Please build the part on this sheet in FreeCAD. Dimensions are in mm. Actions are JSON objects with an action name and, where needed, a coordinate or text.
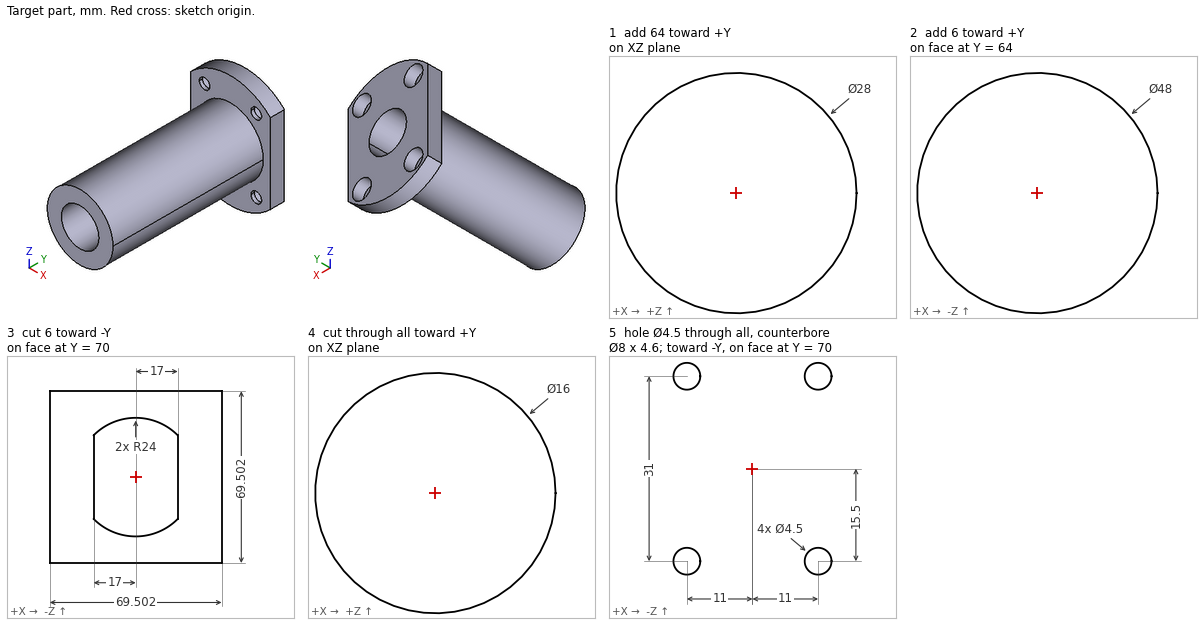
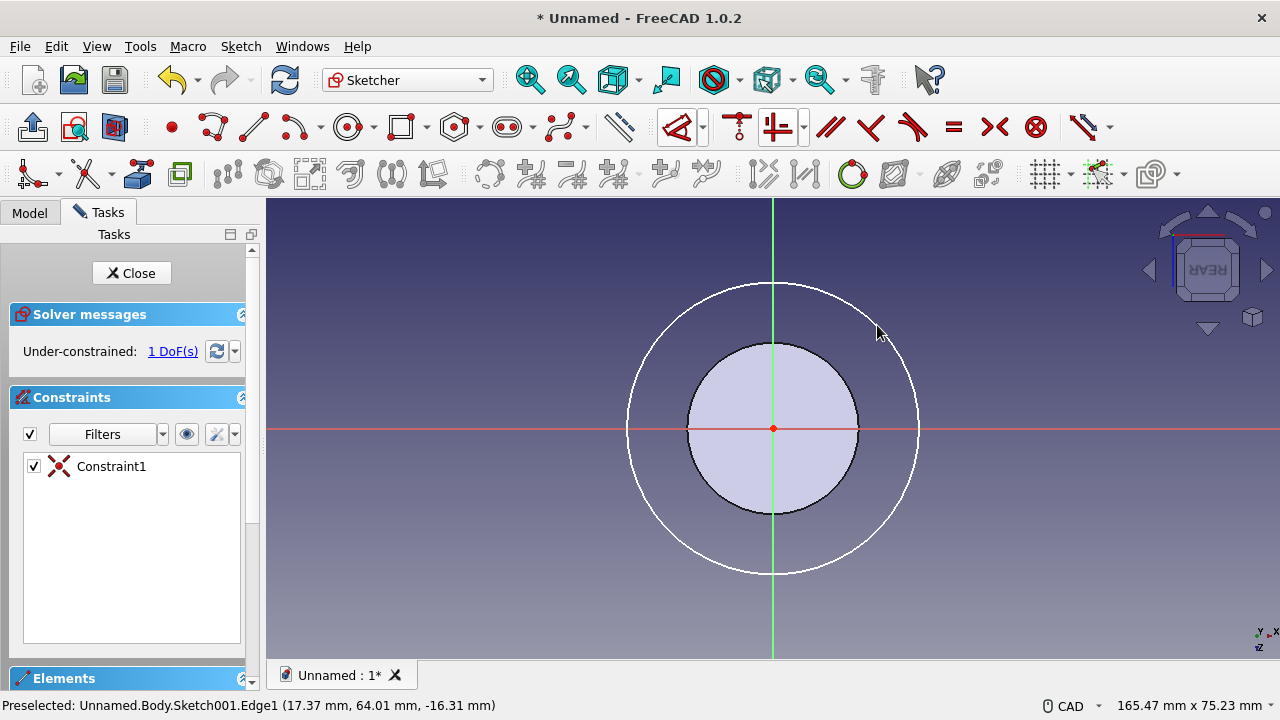
{"action": "left_click", "coordinate": [876, 325]}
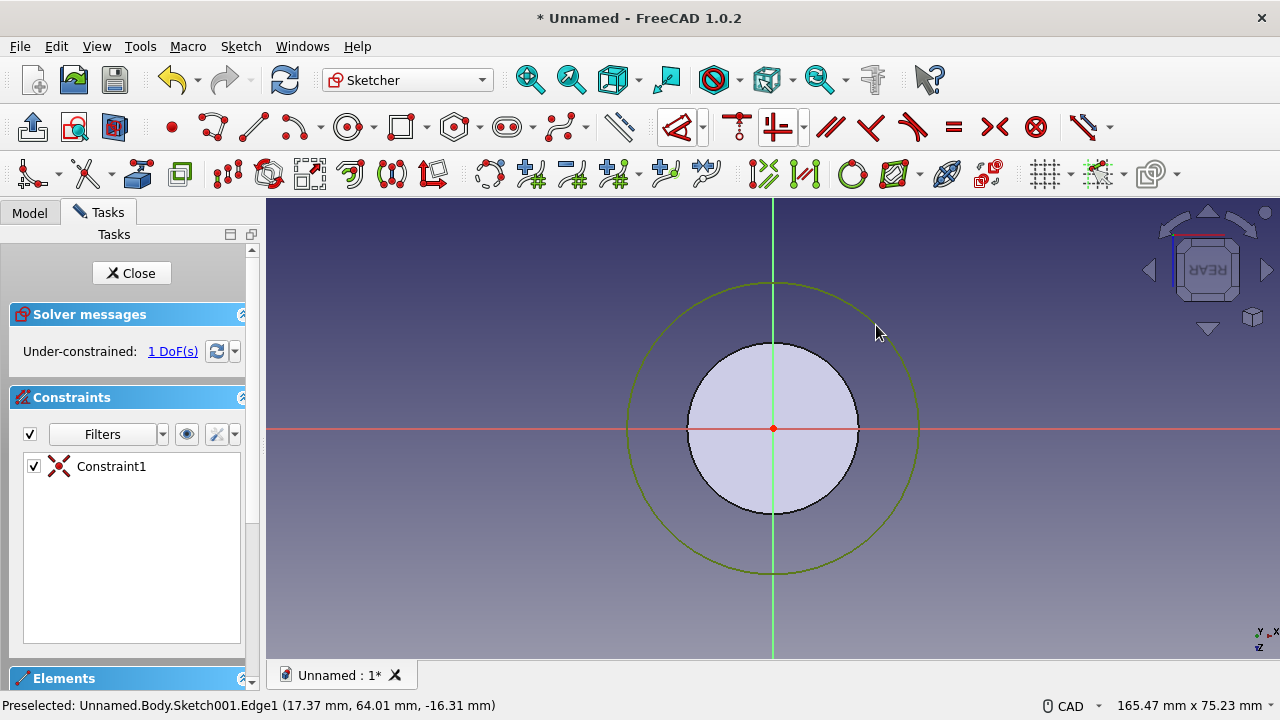
{"action": "key", "text": "k o"}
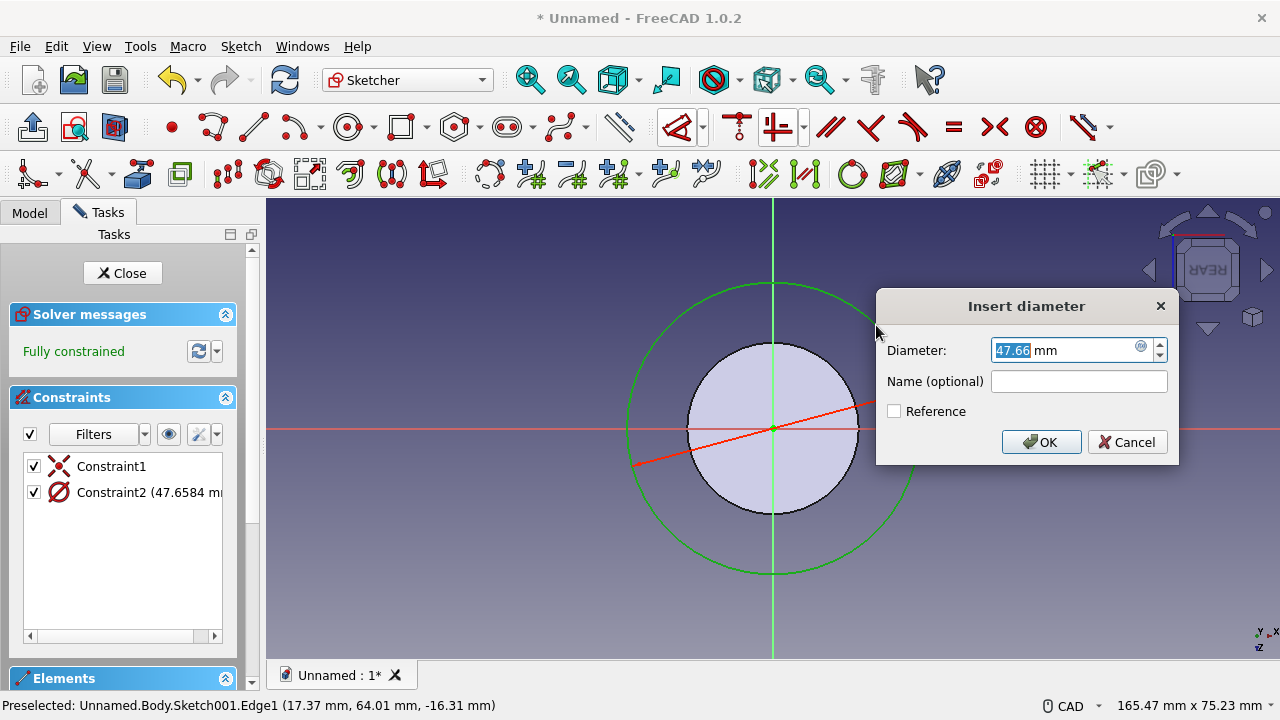
{"action": "type", "text": "48"}
{"action": "key", "text": "Return"}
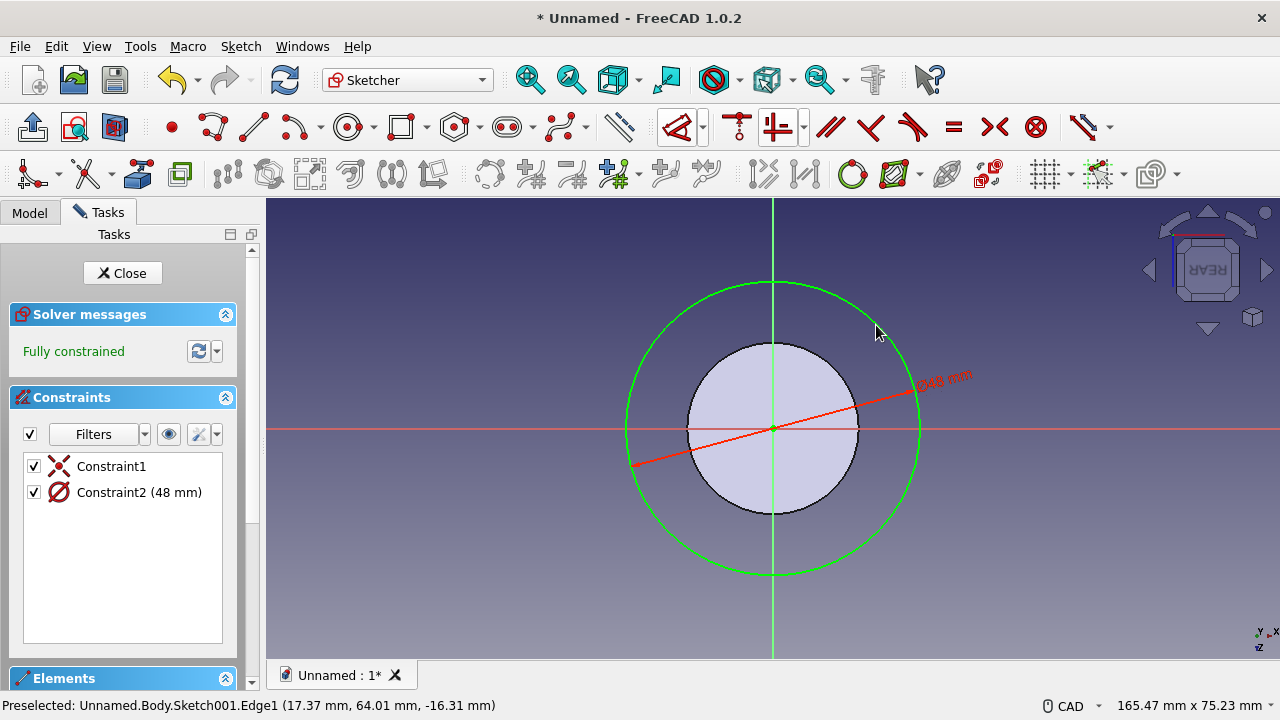
{"action": "left_click", "coordinate": [123, 273]}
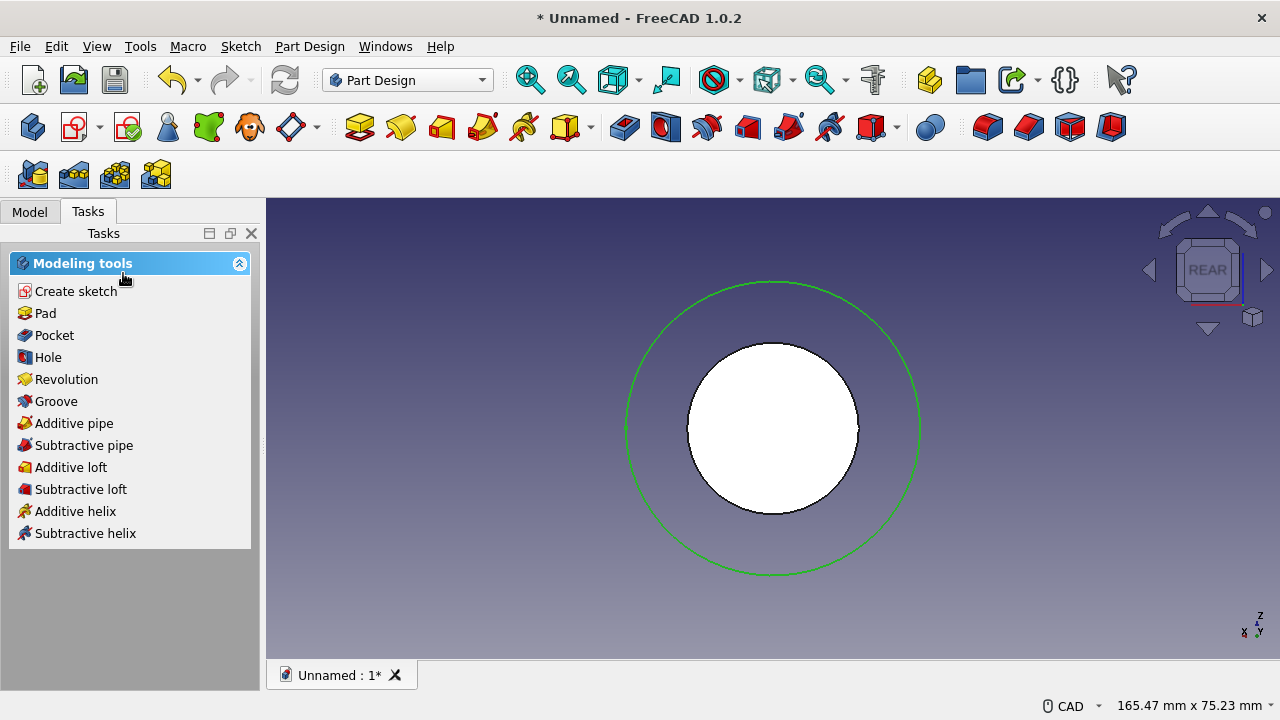
{"action": "left_click", "coordinate": [360, 128]}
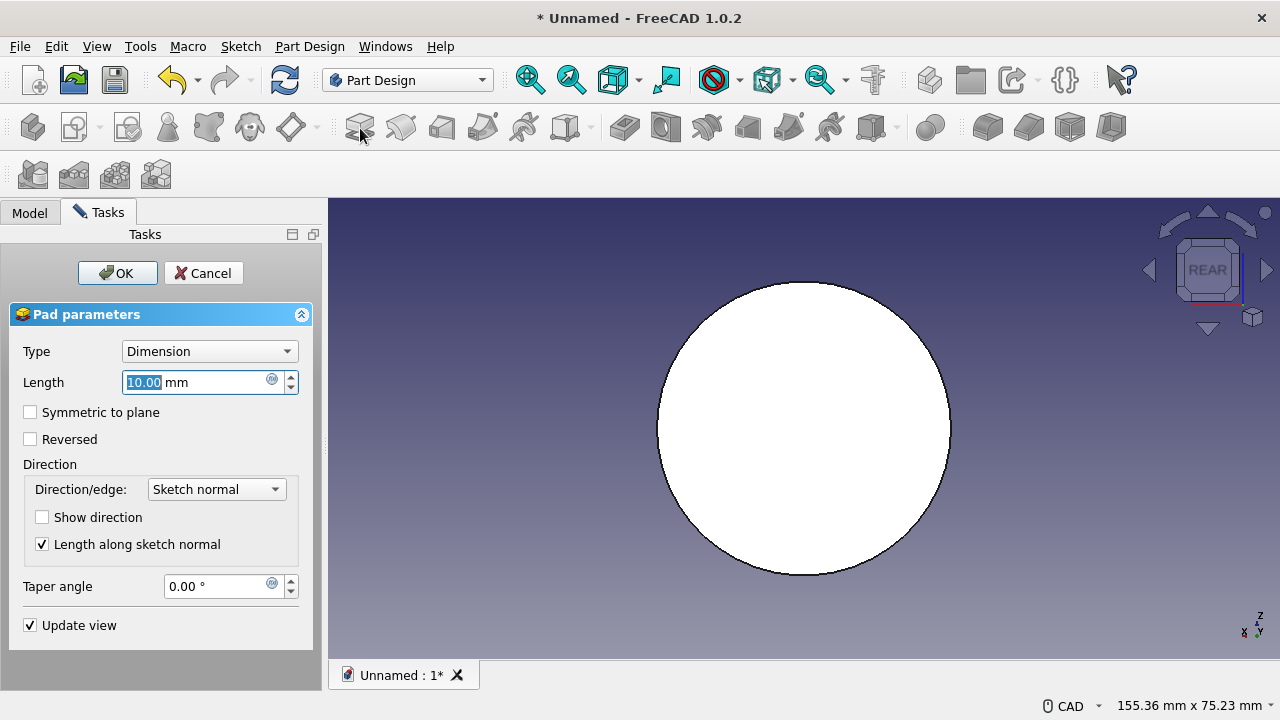
{"action": "type", "text": "6"}
{"action": "key", "text": "Tab"}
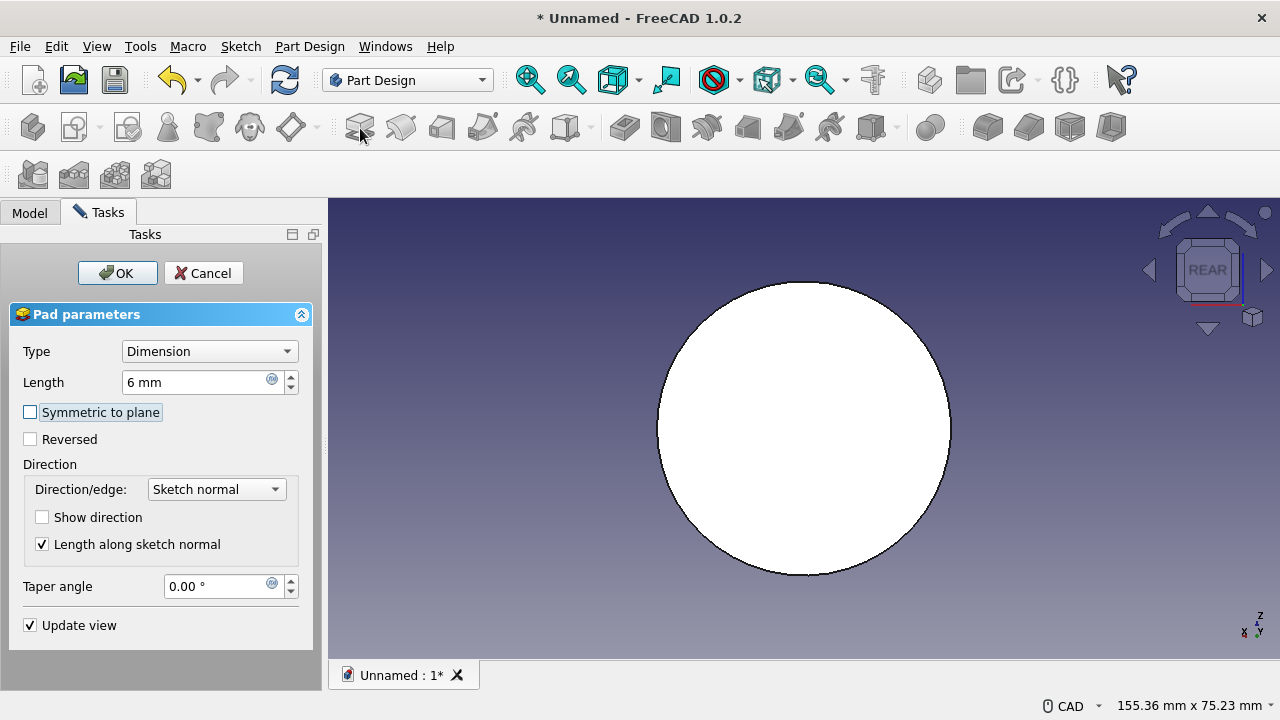
{"action": "left_click", "coordinate": [118, 273]}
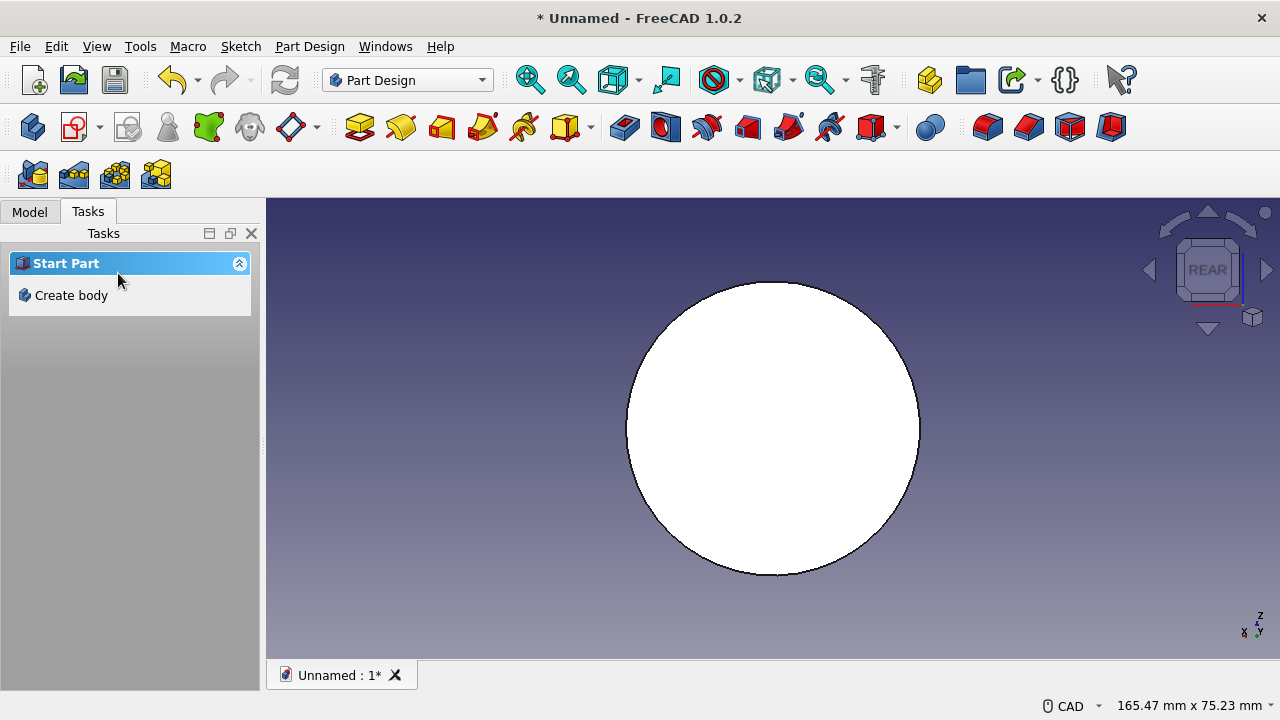
{"action": "left_click", "coordinate": [773, 428]}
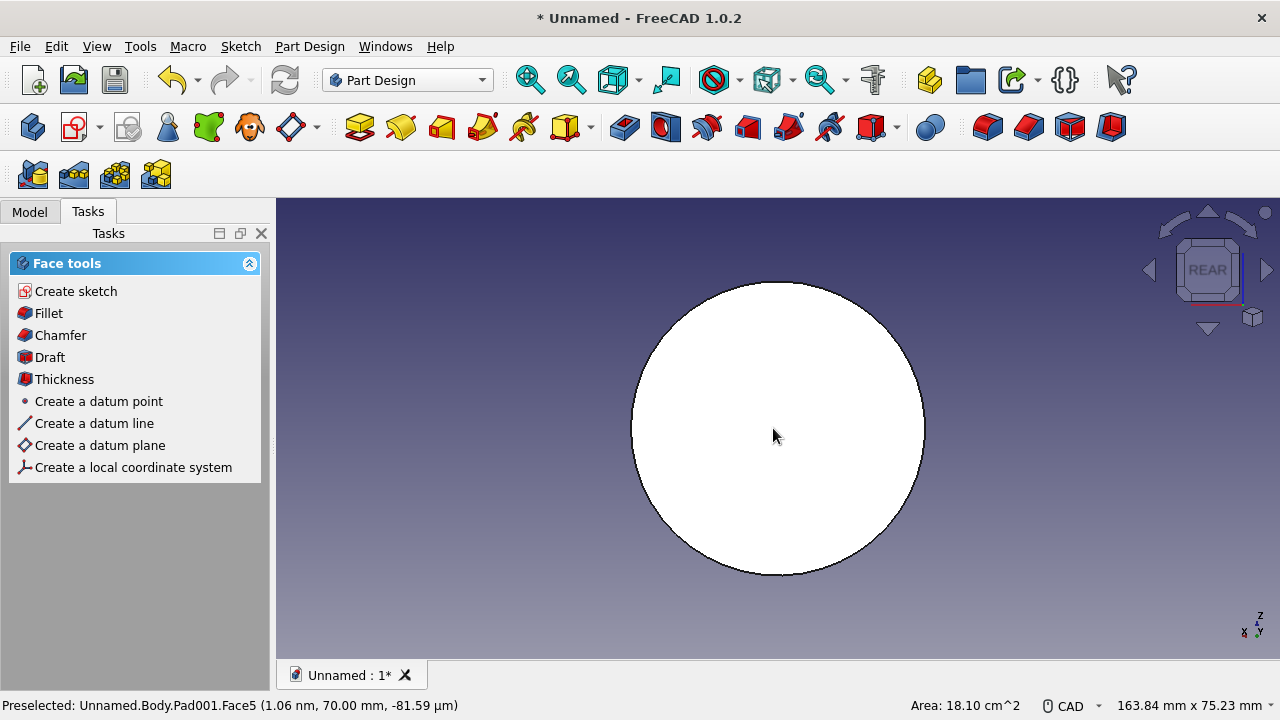
{"action": "left_click", "coordinate": [74, 128]}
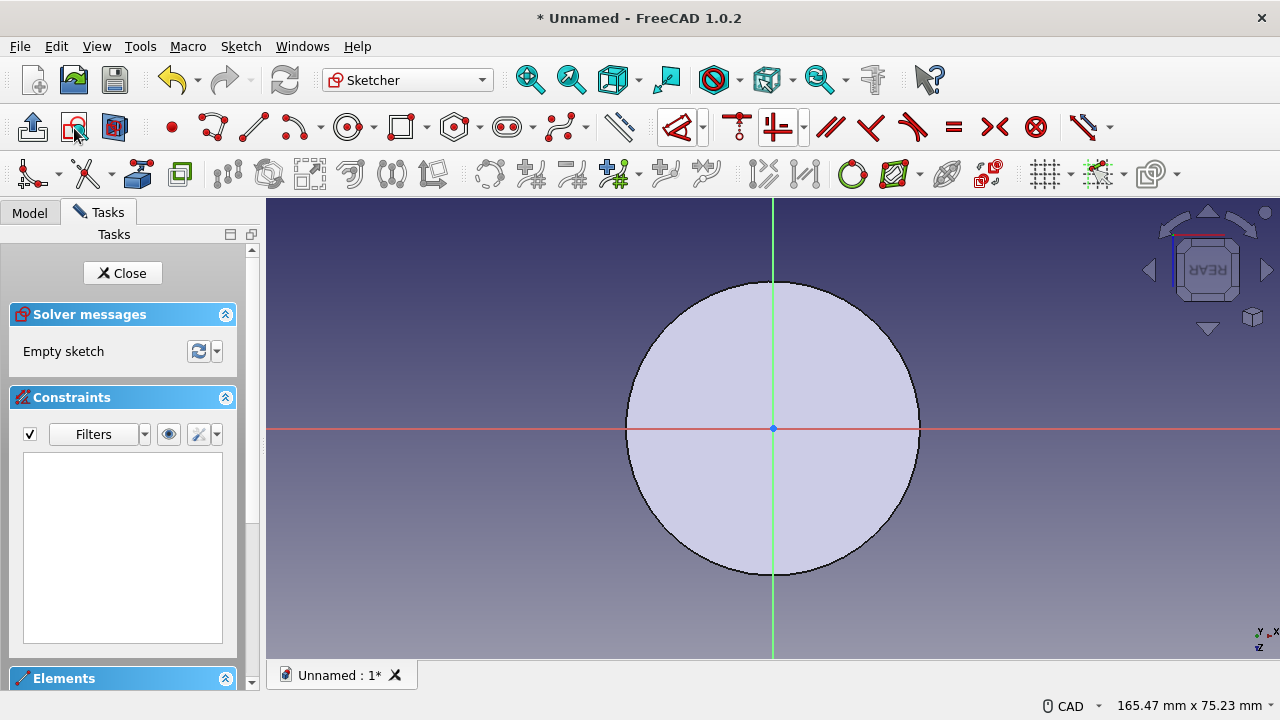
{"action": "scroll", "coordinate": [565, 429], "scroll_direction": "down", "scroll_amount": 2}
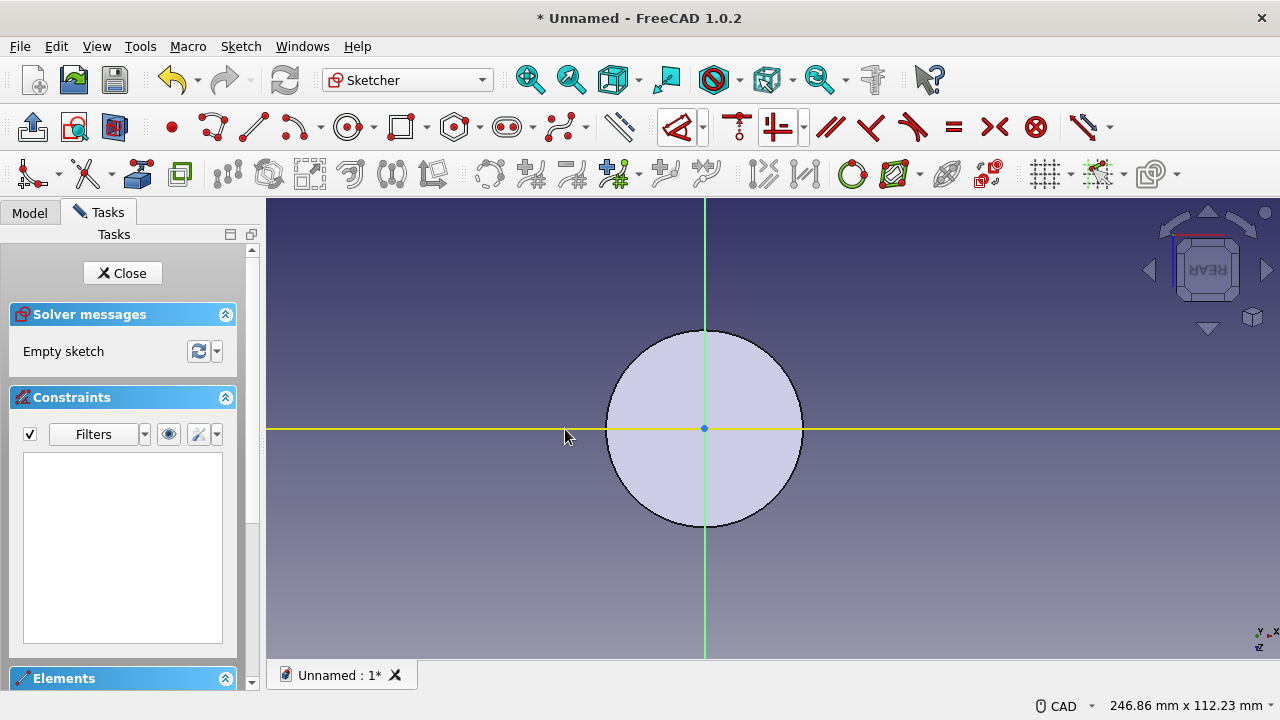
{"action": "left_click", "coordinate": [426, 128]}